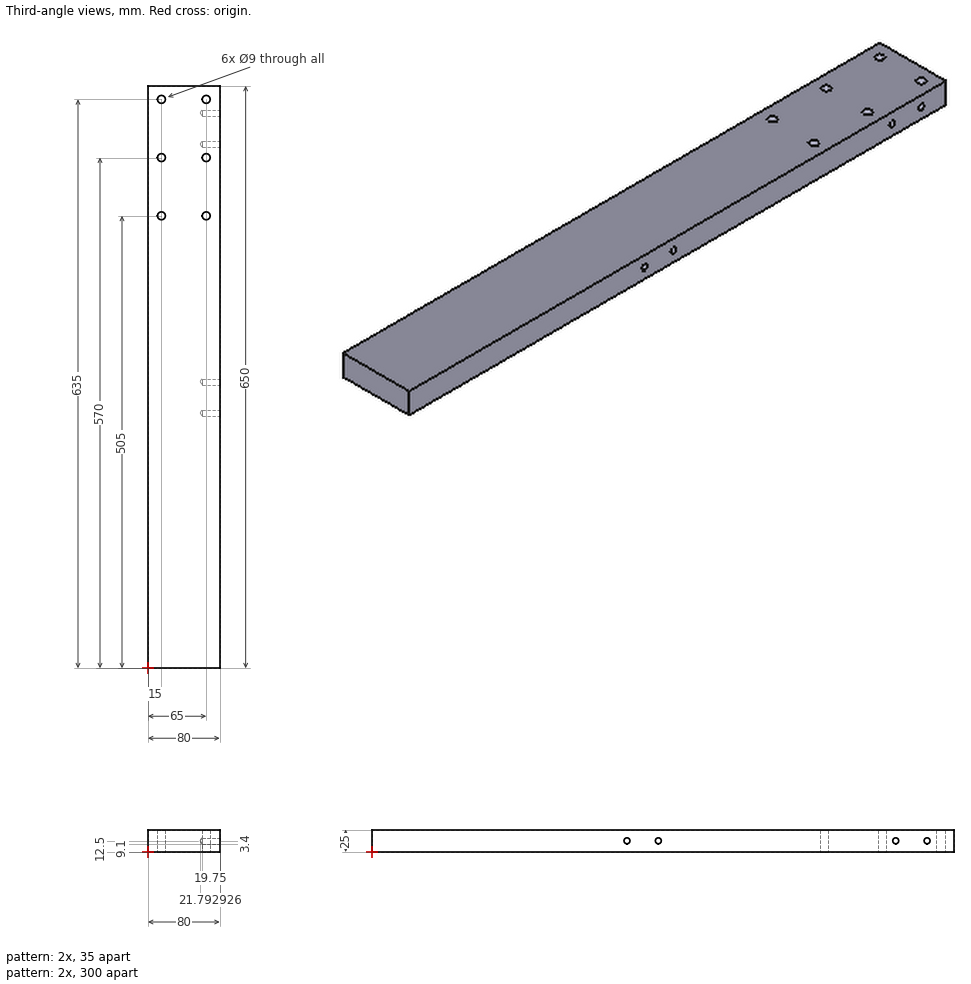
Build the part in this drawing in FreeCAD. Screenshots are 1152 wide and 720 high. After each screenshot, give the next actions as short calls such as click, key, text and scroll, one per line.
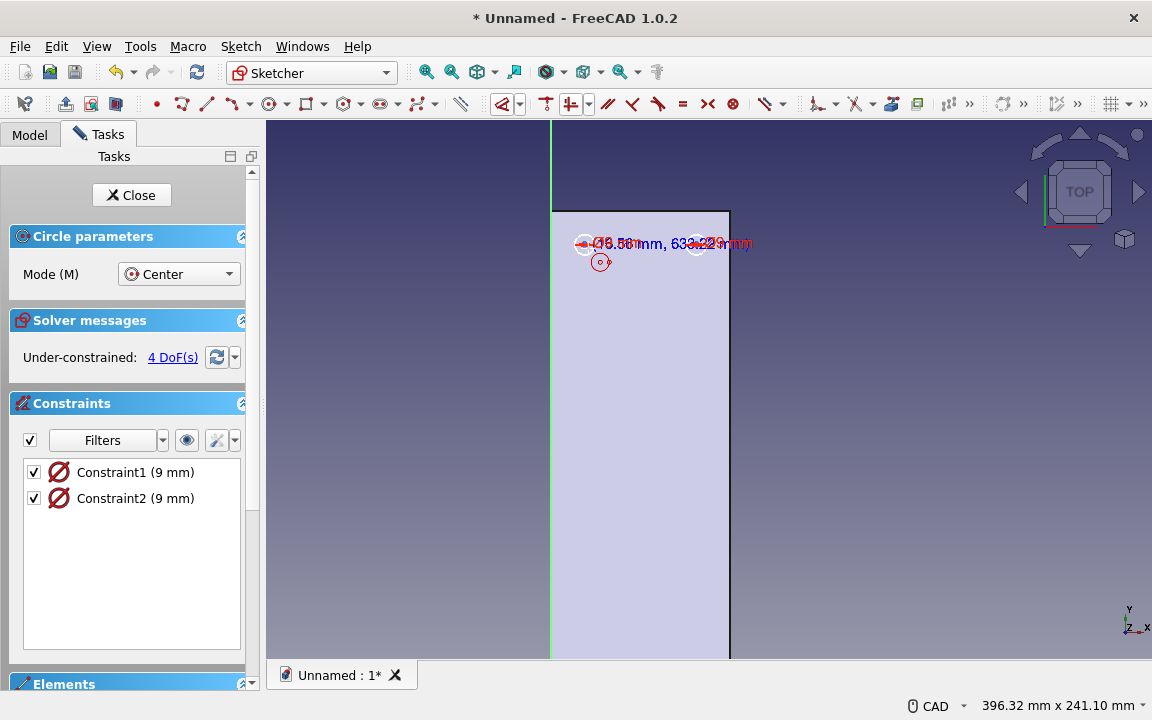
scroll(585, 535, up, 5)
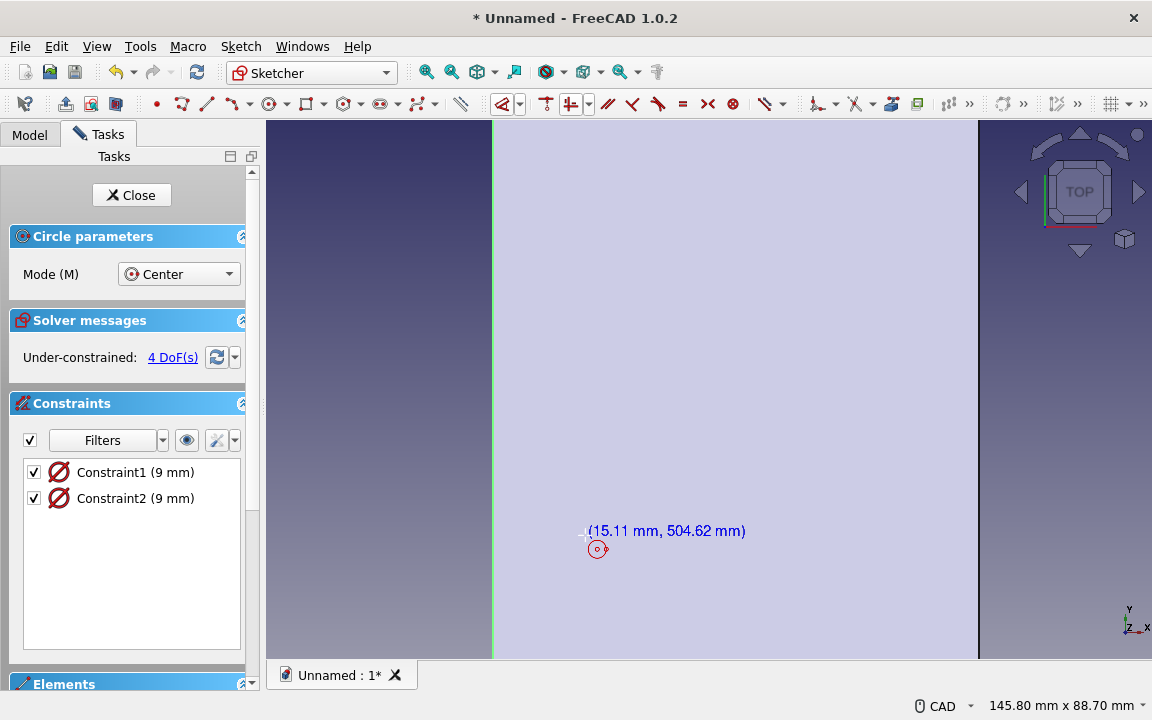
click(584, 534)
move(603, 515)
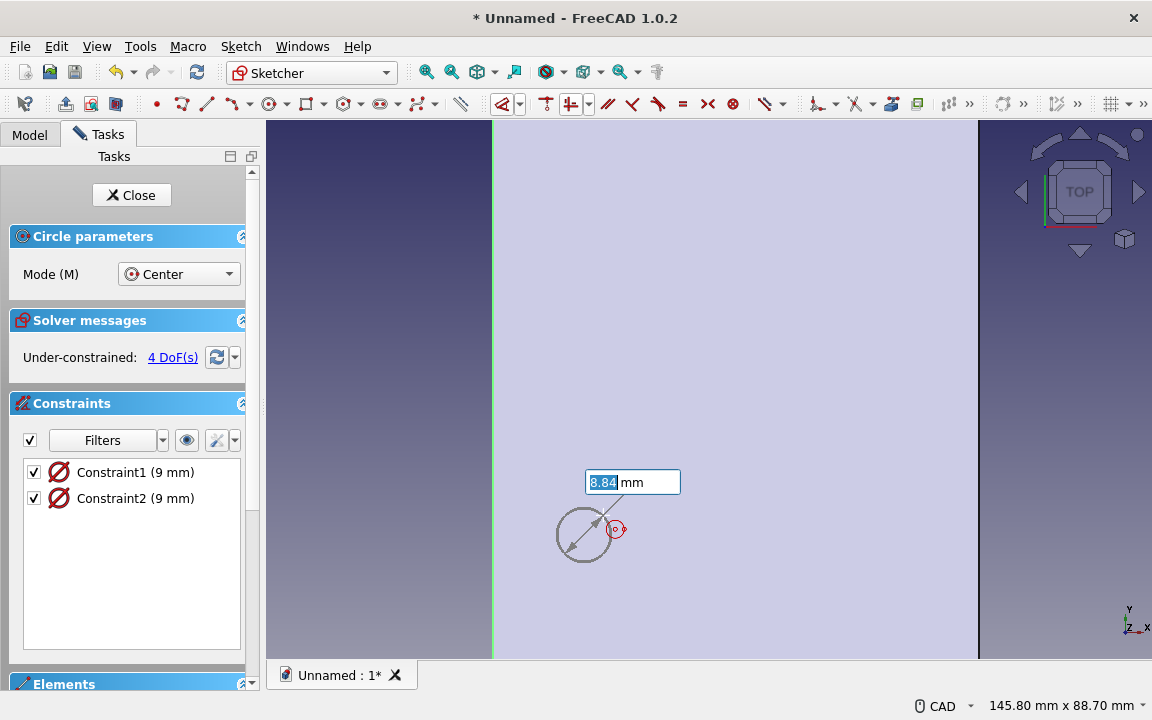
text(9)
key(Return)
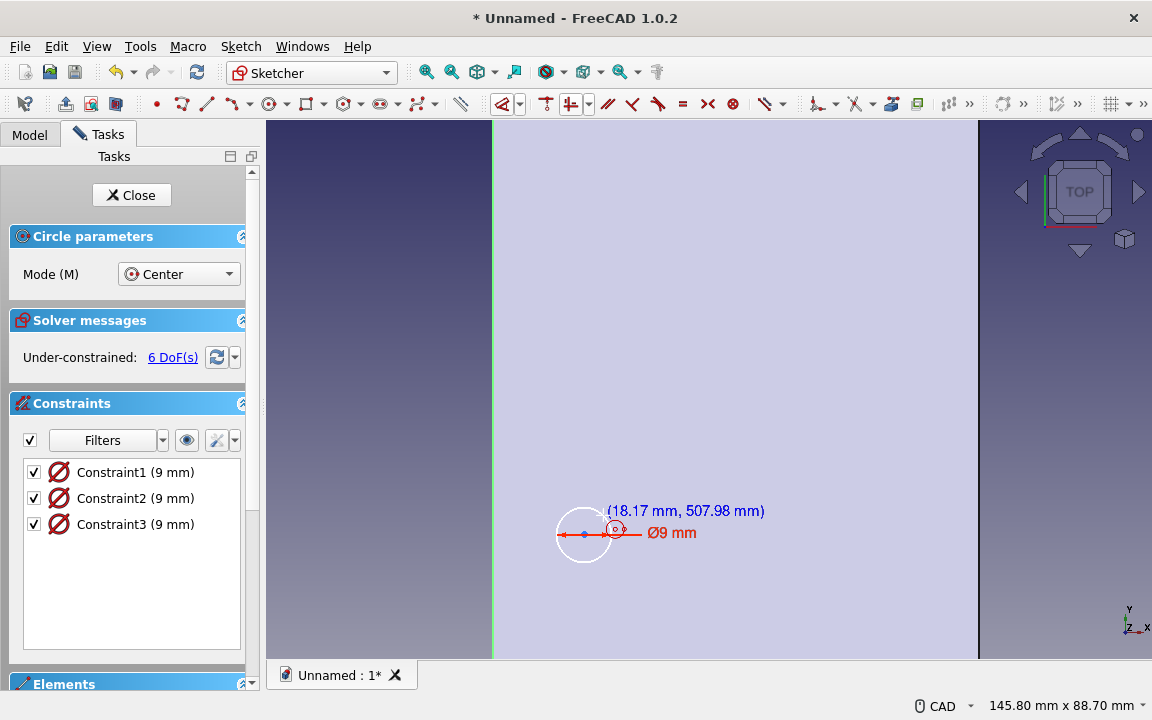
click(888, 534)
move(907, 515)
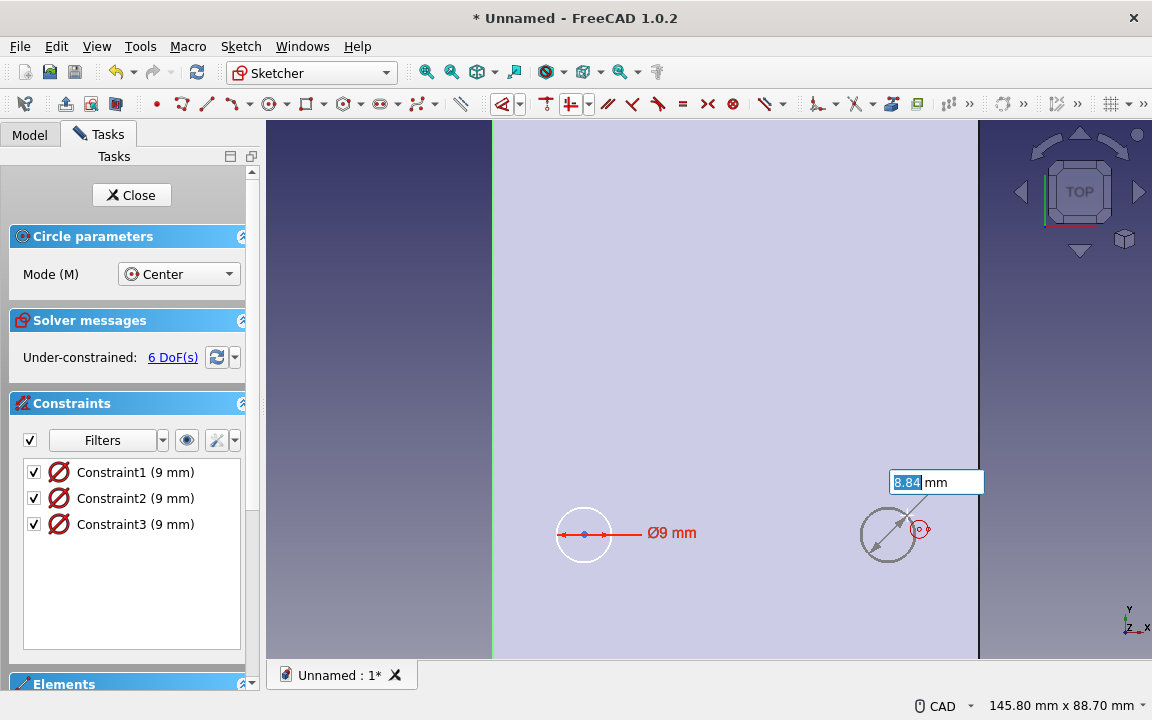
text(9)
key(Return)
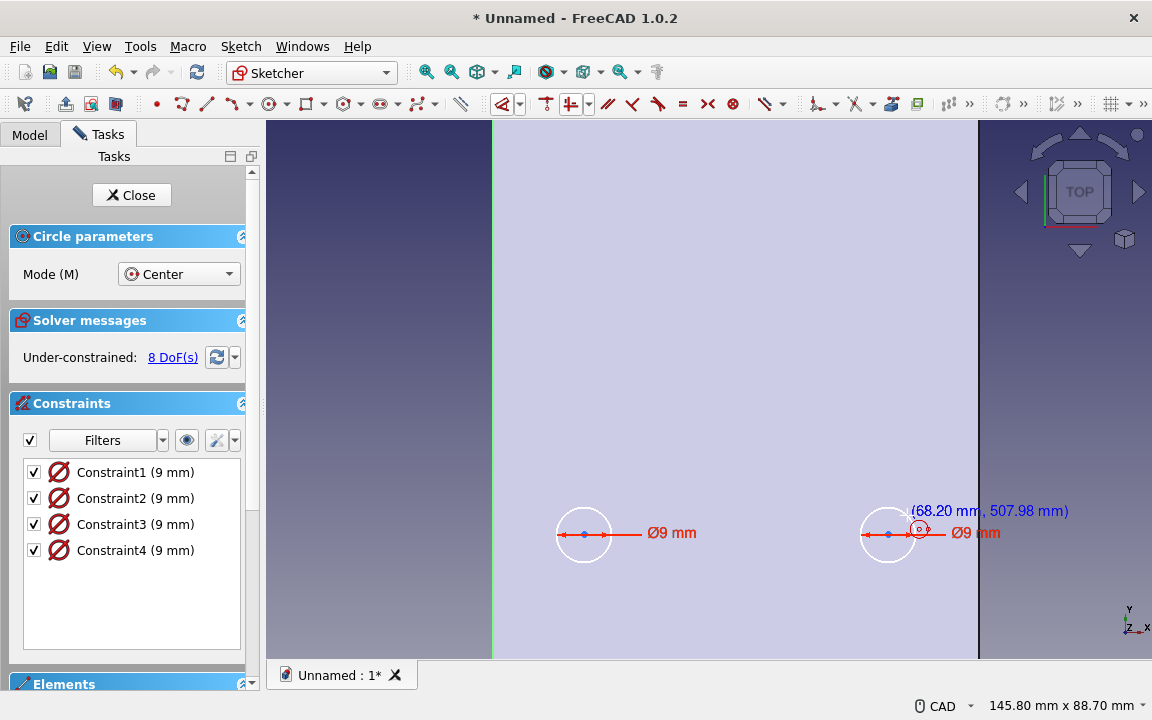
scroll(585, 535, down, 5)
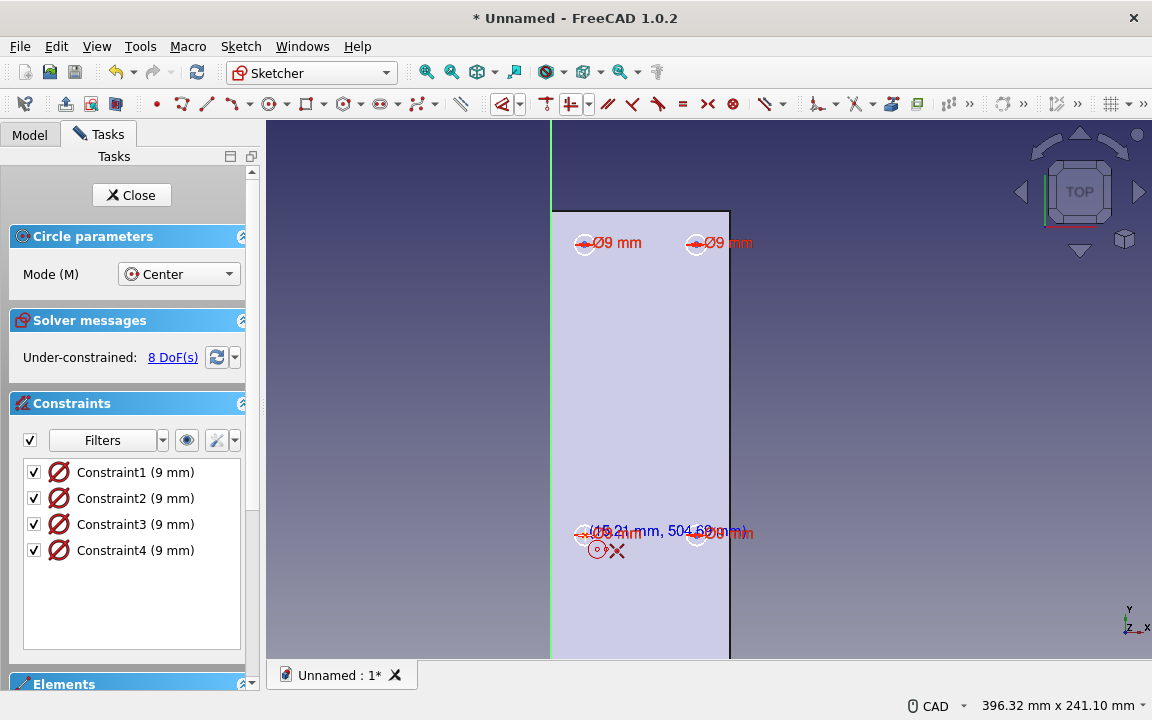
scroll(585, 390, up, 5)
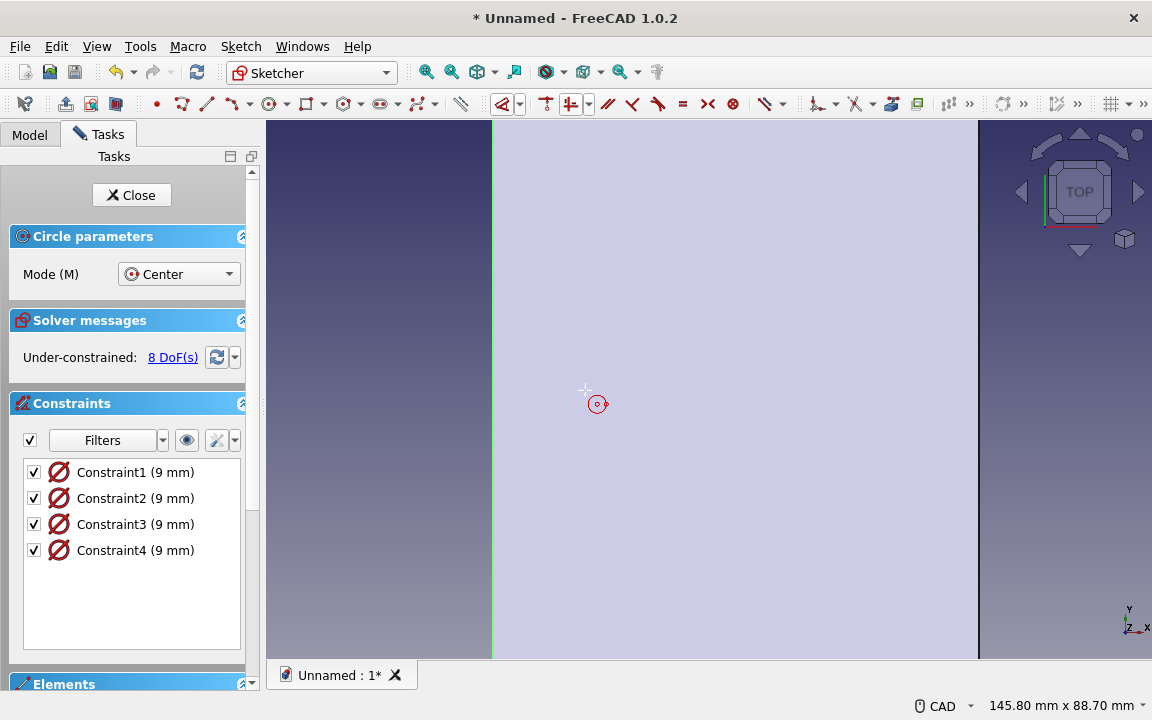
click(584, 389)
move(603, 369)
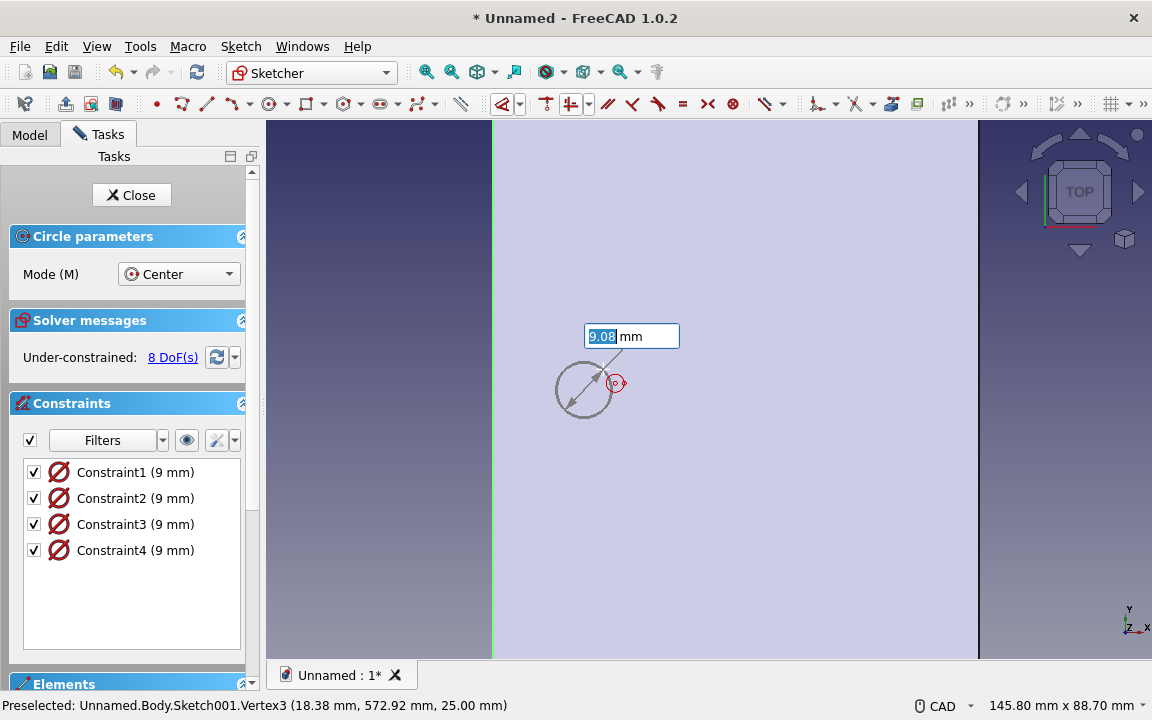
text(9)
key(Return)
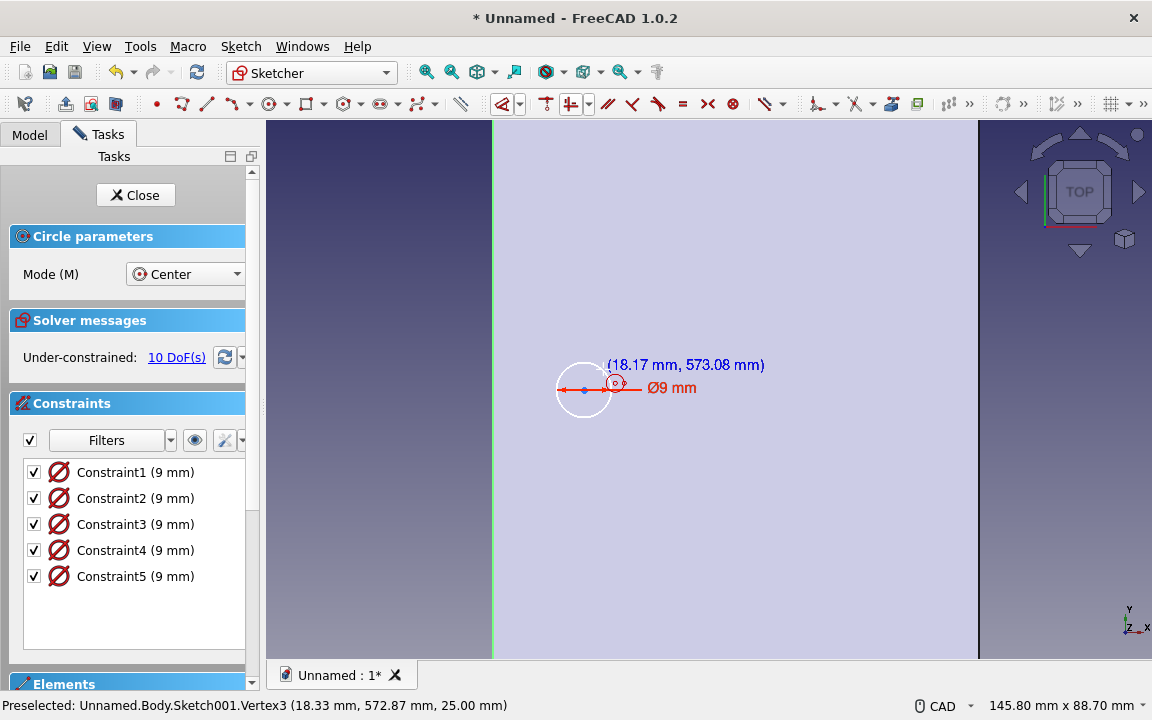
click(888, 389)
move(907, 369)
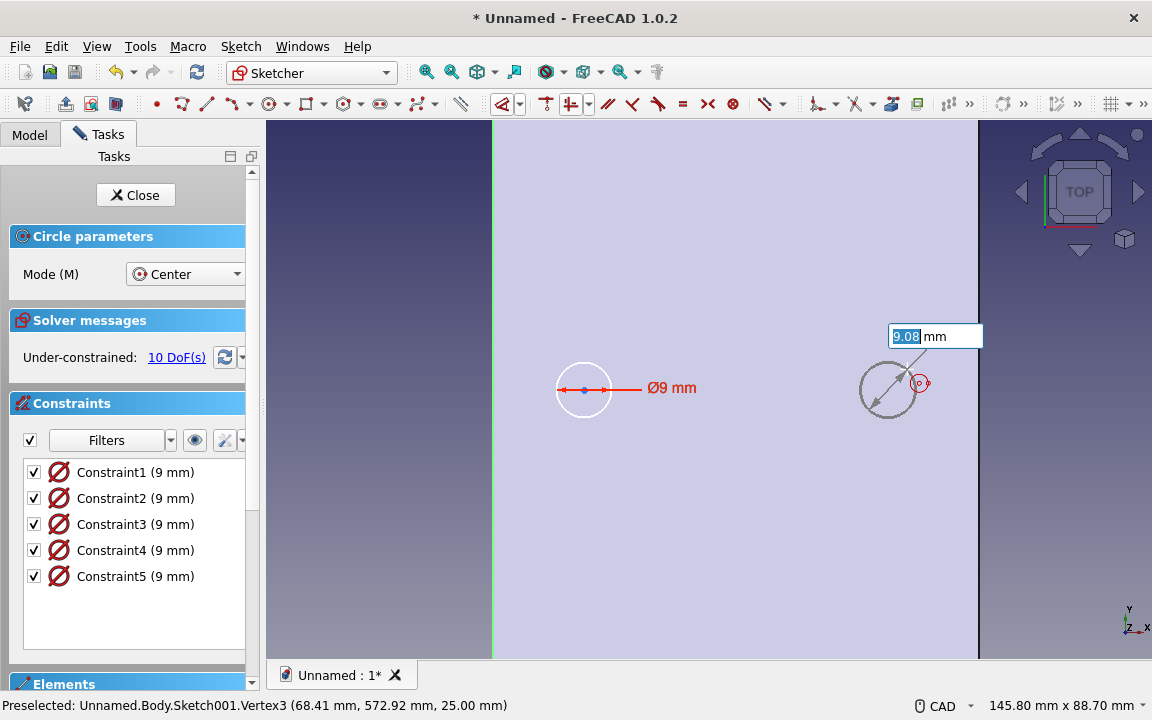
text(9)
key(Return)
key(Escape)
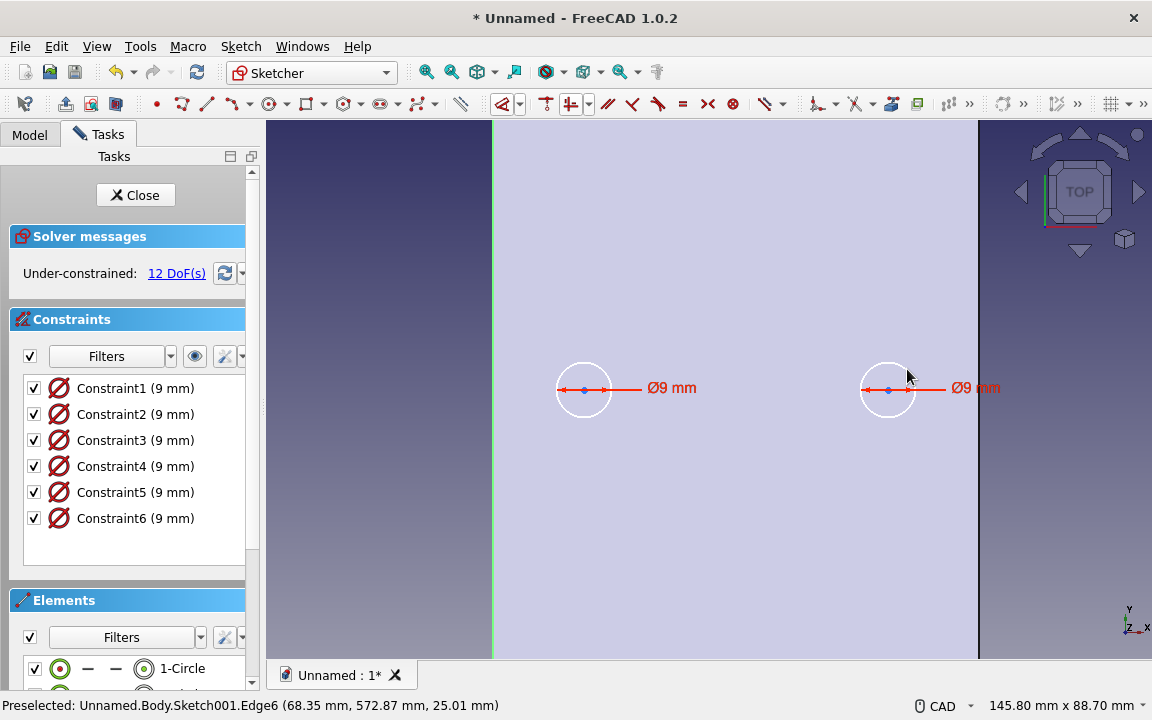
scroll(585, 390, down, 5)